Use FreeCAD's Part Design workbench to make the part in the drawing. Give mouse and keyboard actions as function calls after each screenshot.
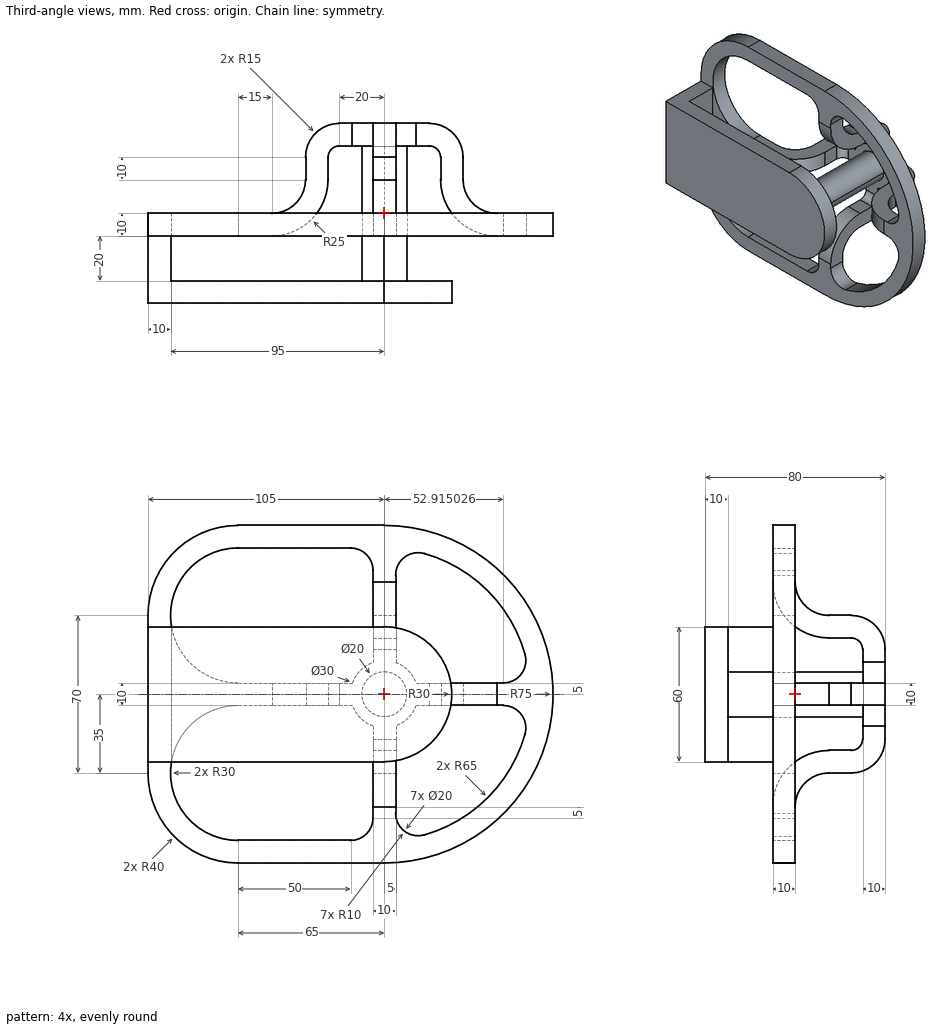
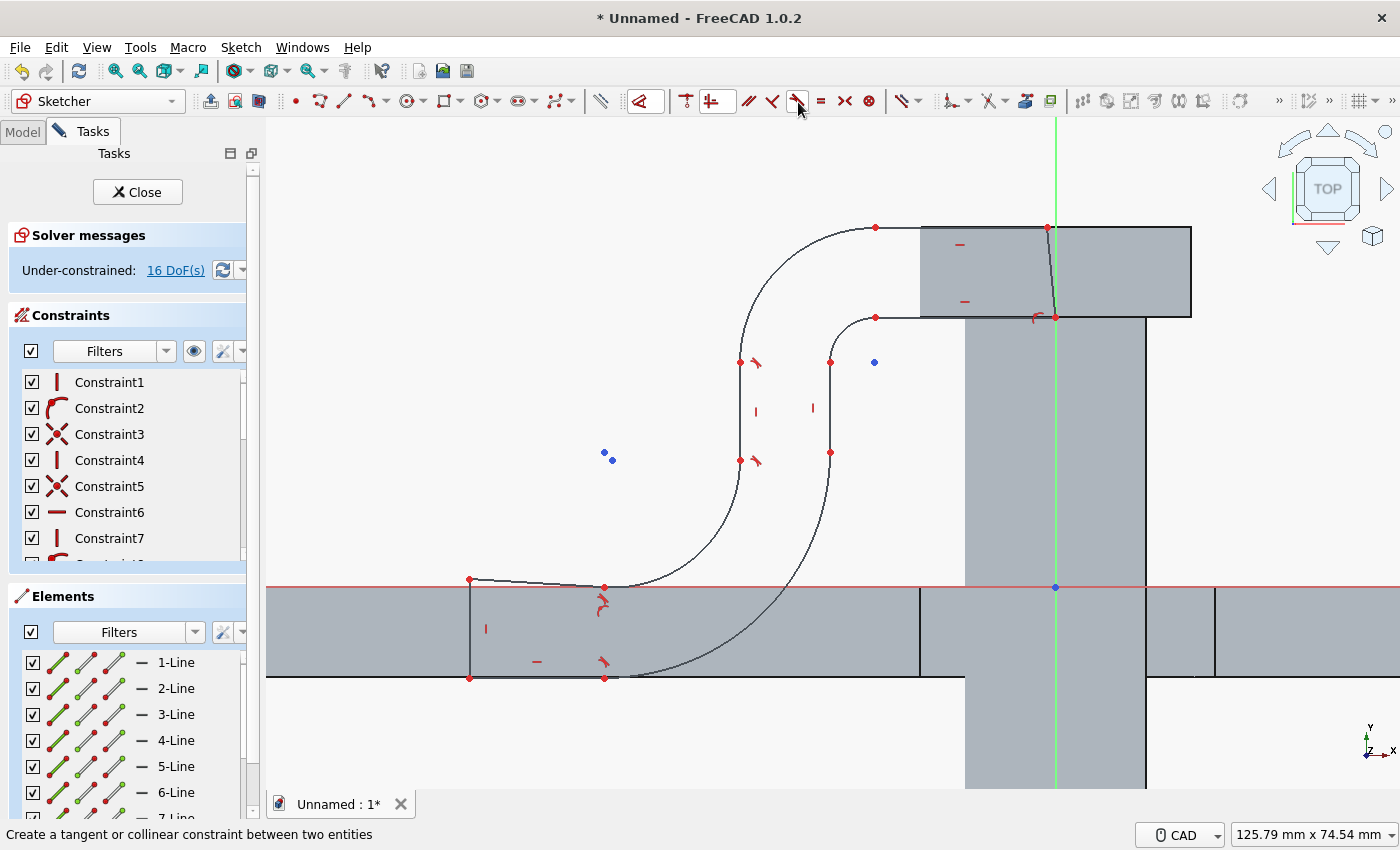
click(830, 426)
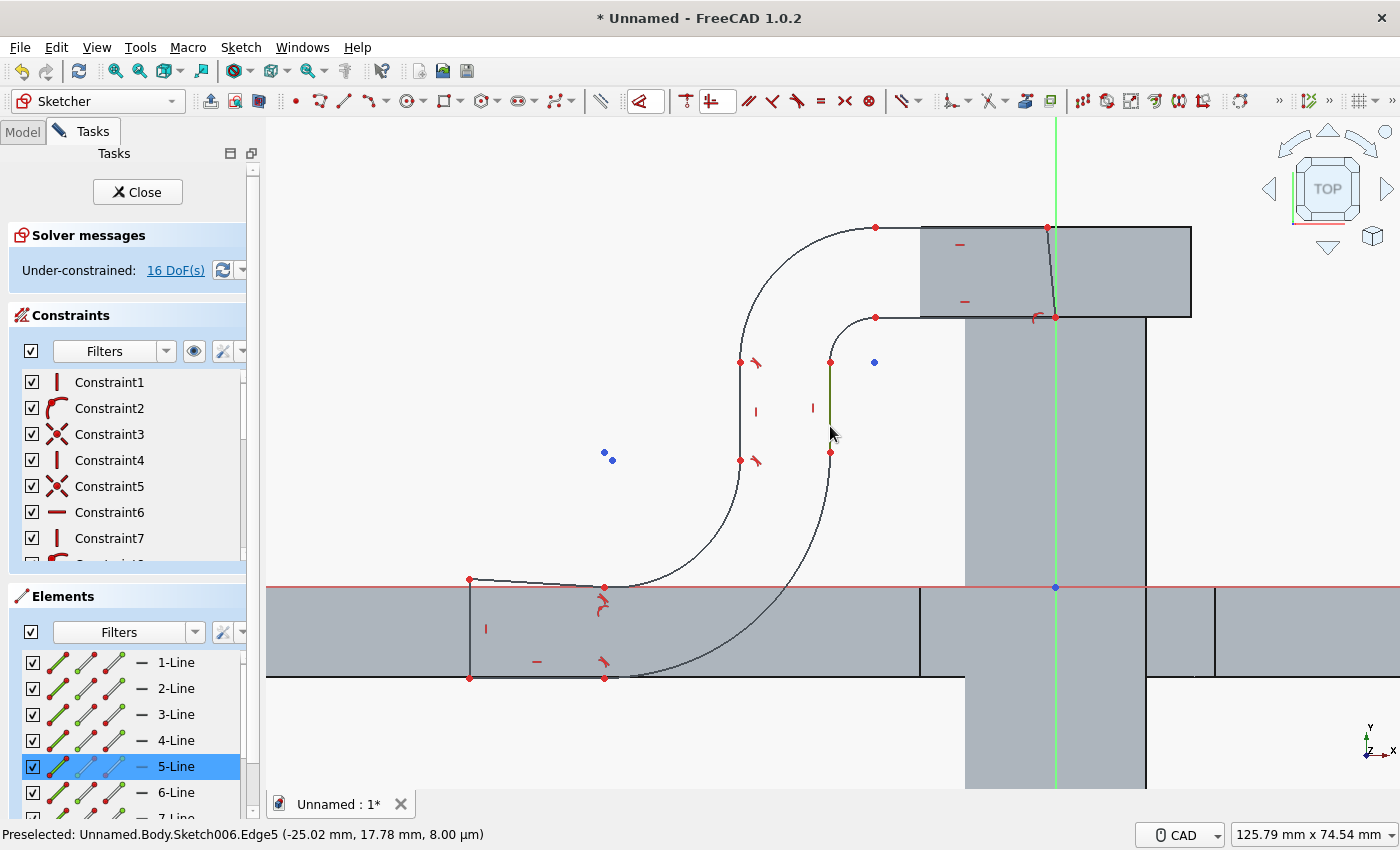
click(707, 653)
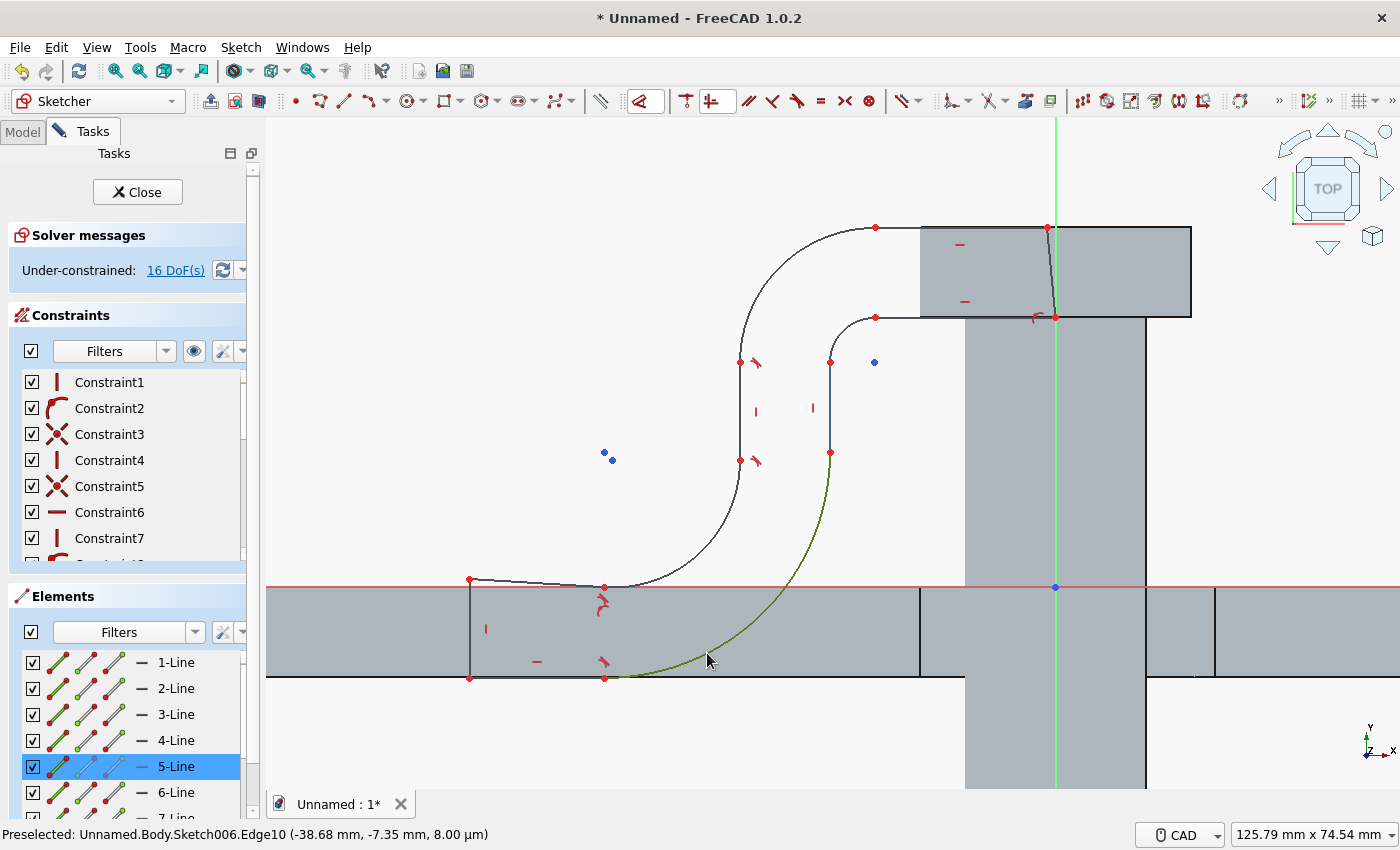
click(798, 102)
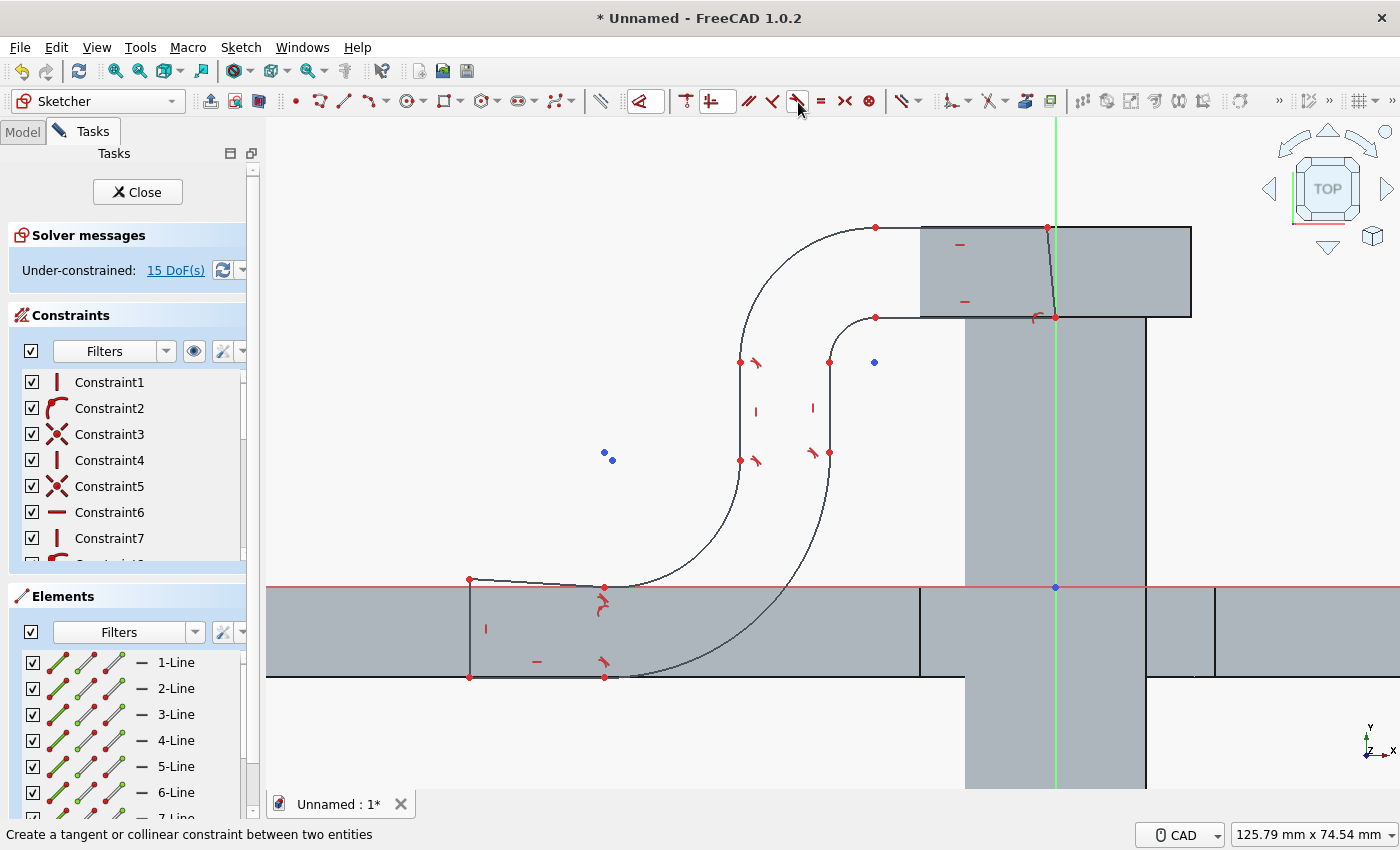
click(830, 426)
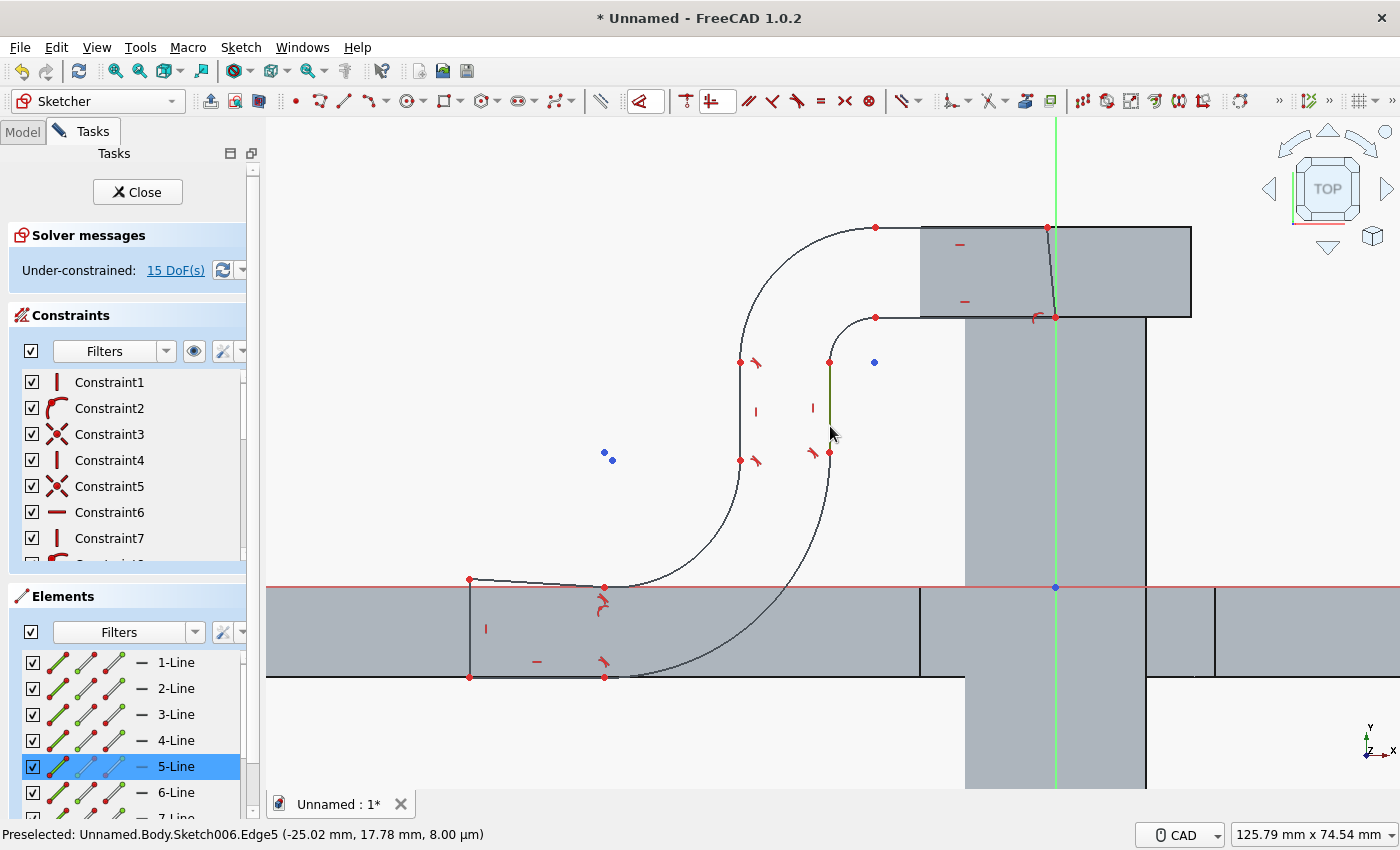
click(854, 323)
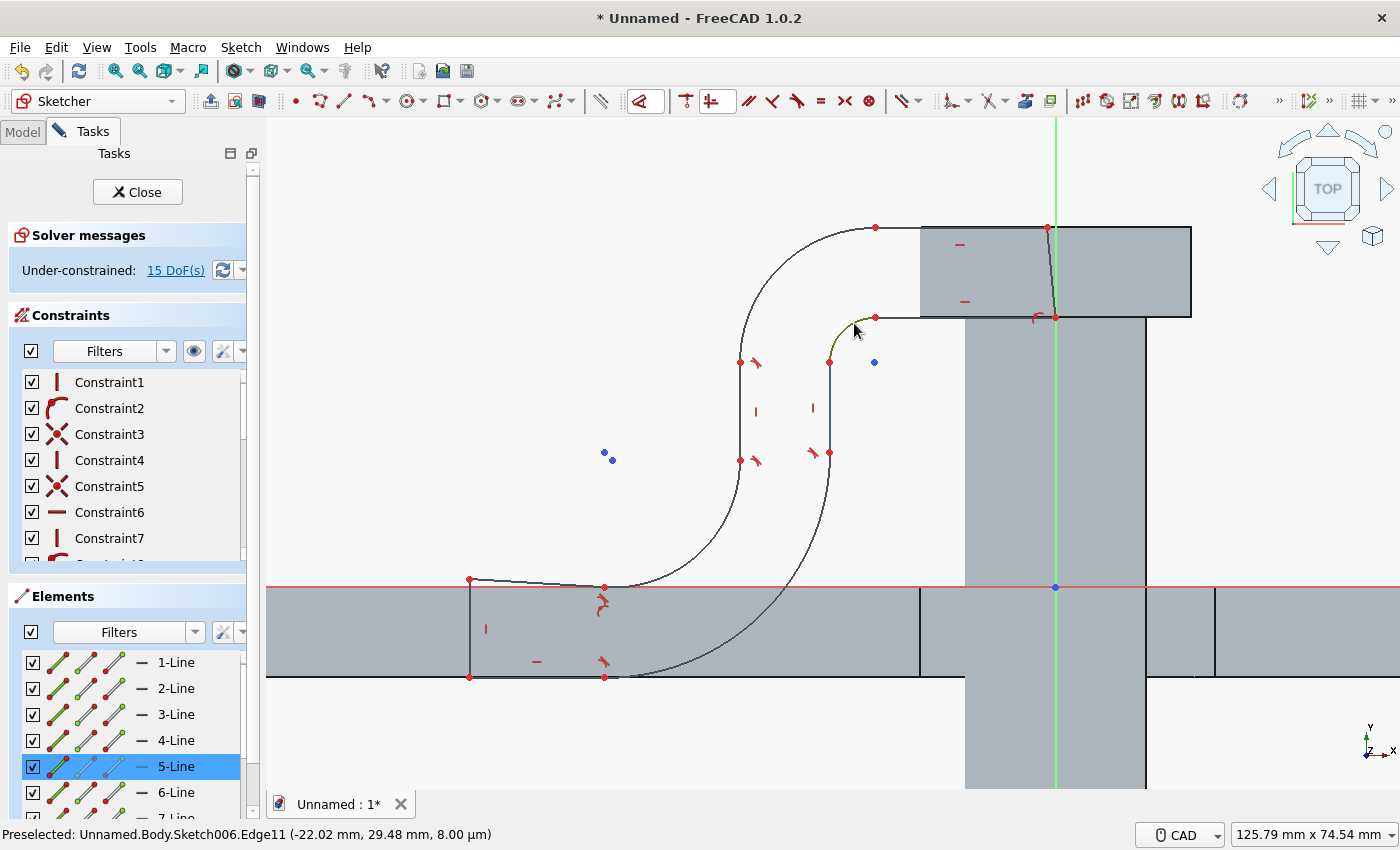
click(798, 102)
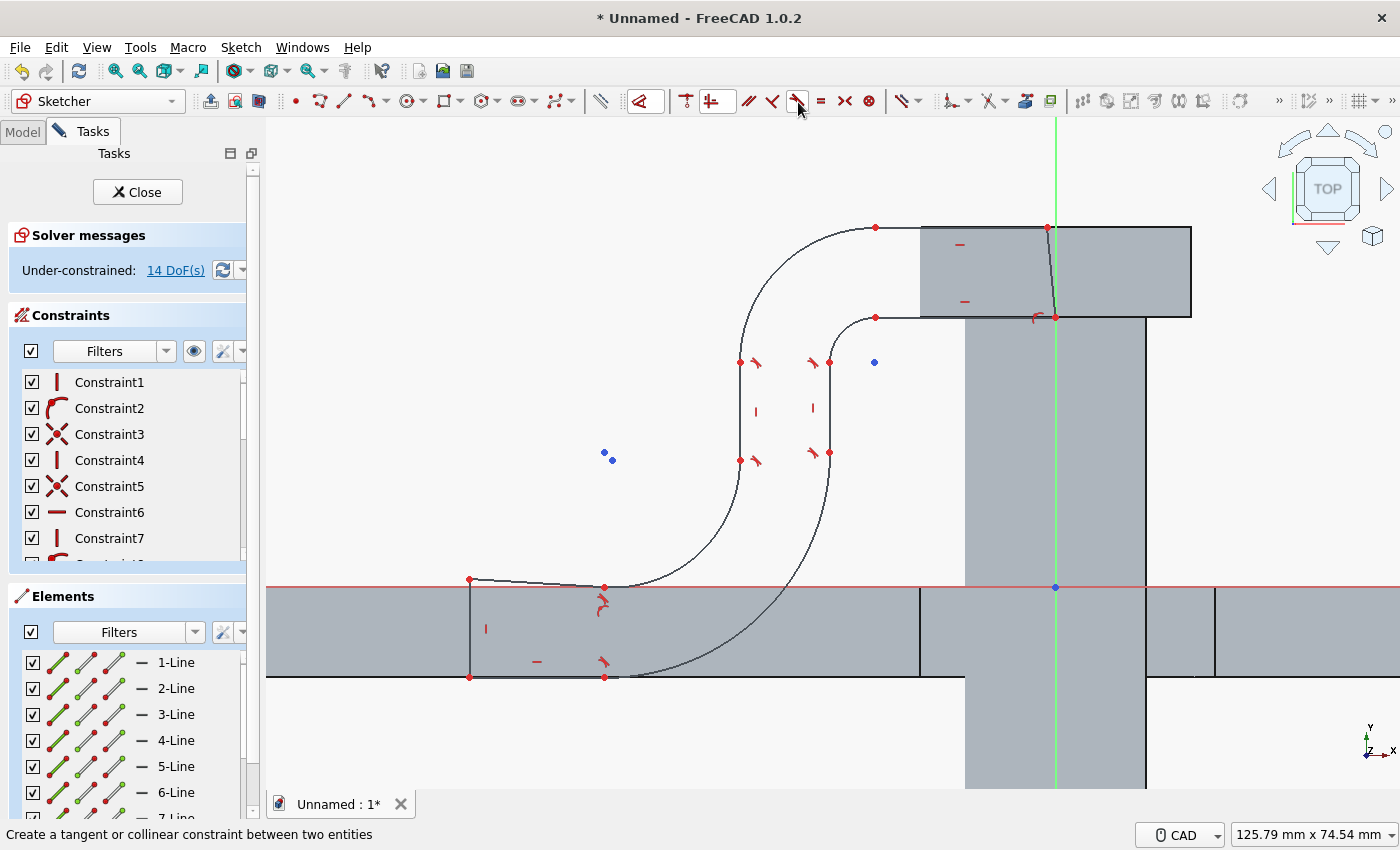
click(929, 318)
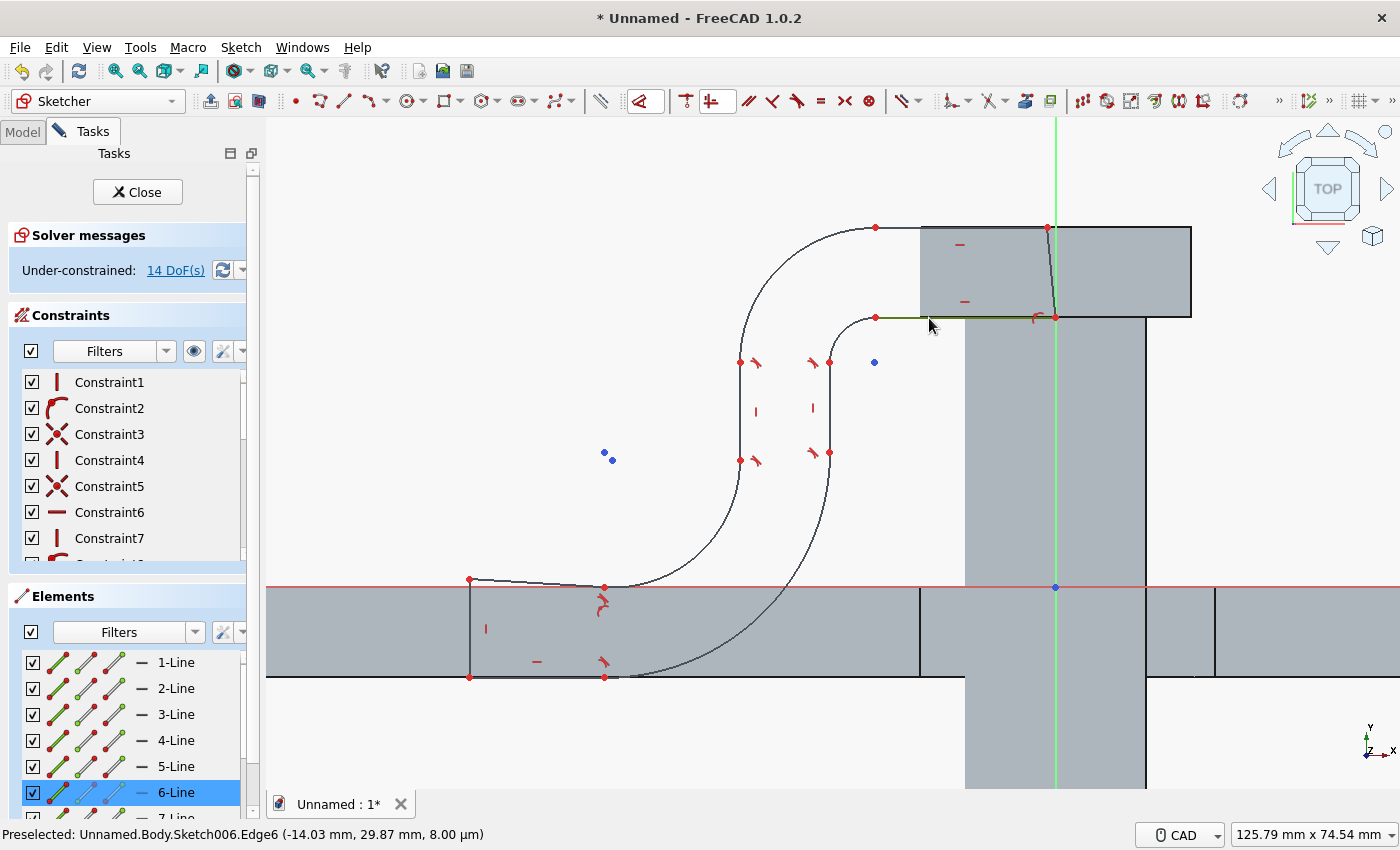
click(855, 323)